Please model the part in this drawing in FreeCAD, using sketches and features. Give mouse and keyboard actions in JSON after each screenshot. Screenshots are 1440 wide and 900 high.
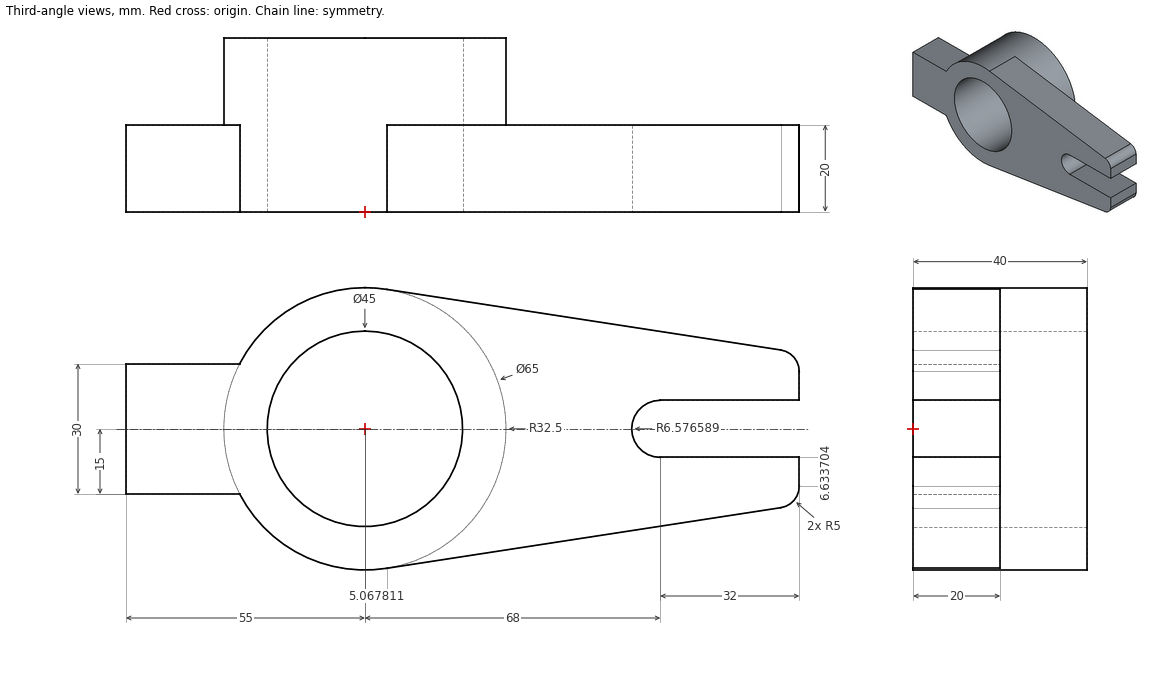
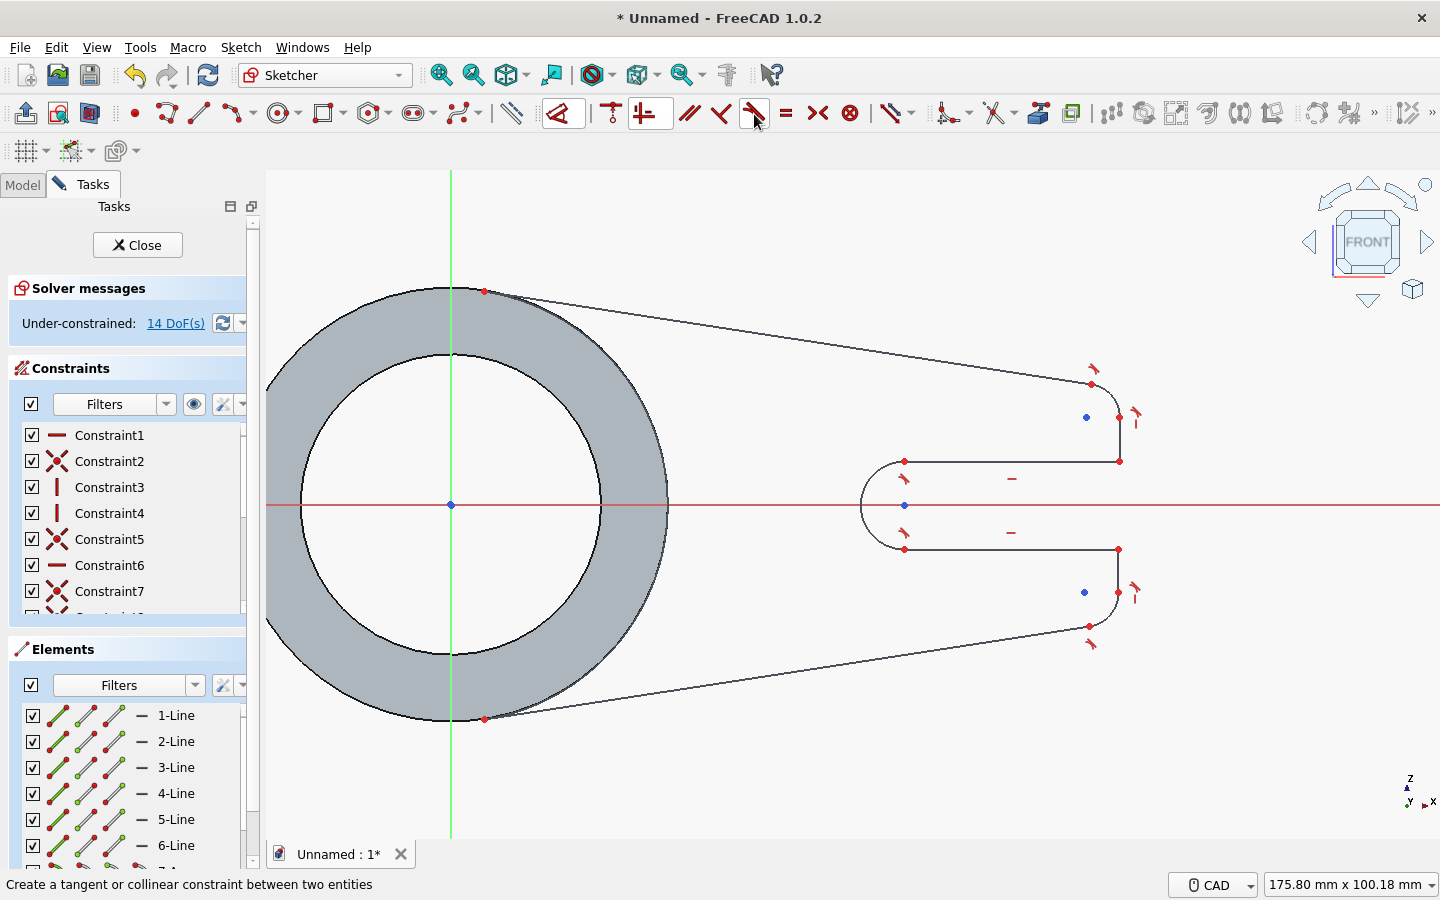
{"action": "left_click_drag", "start_coordinate": [441, 495], "coordinate": [461, 516]}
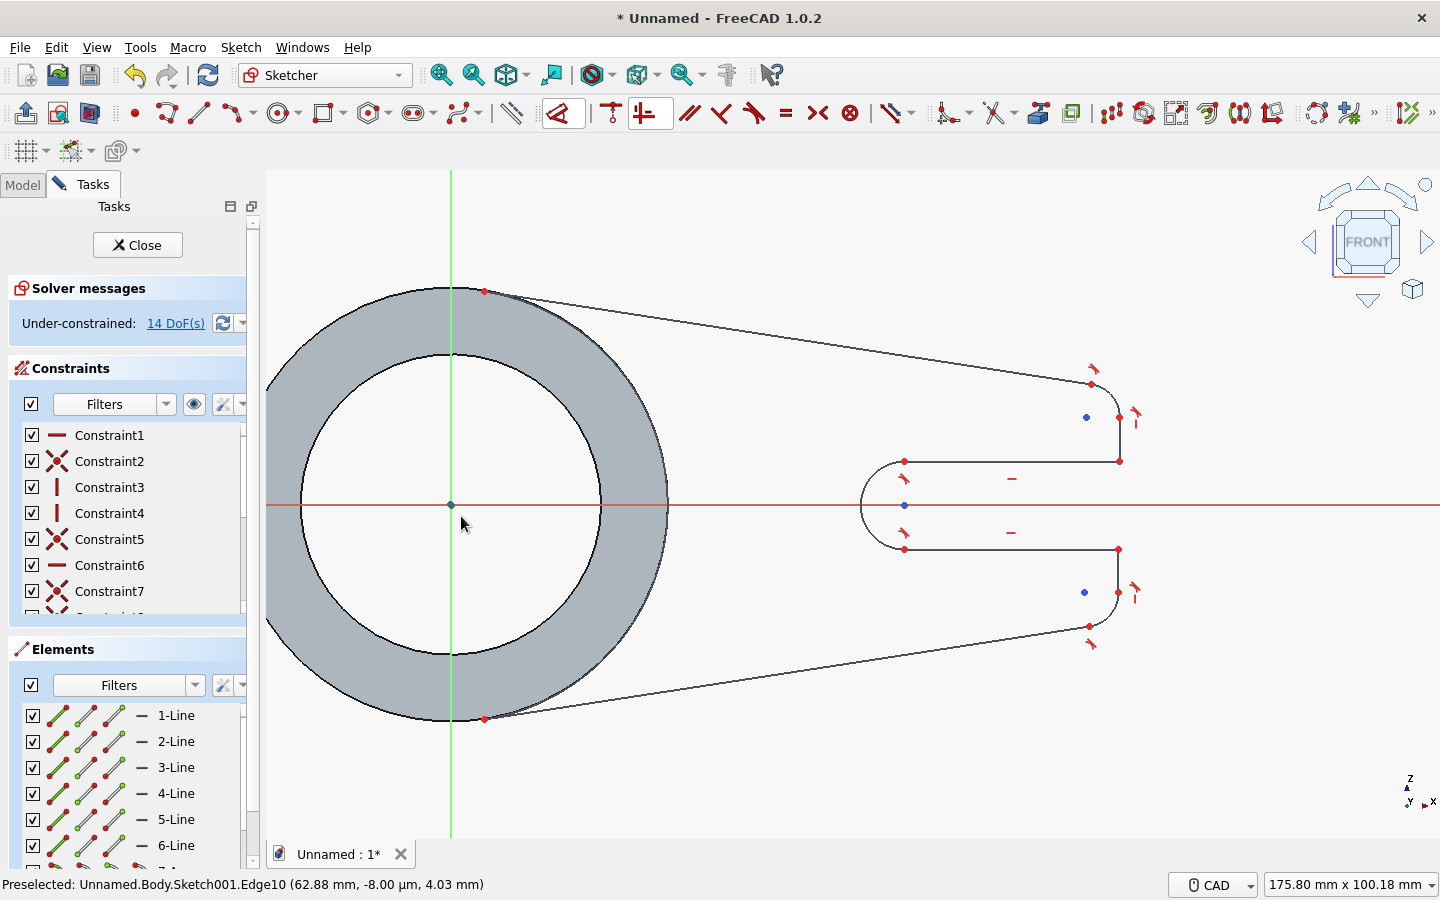
{"action": "left_click", "coordinate": [612, 114]}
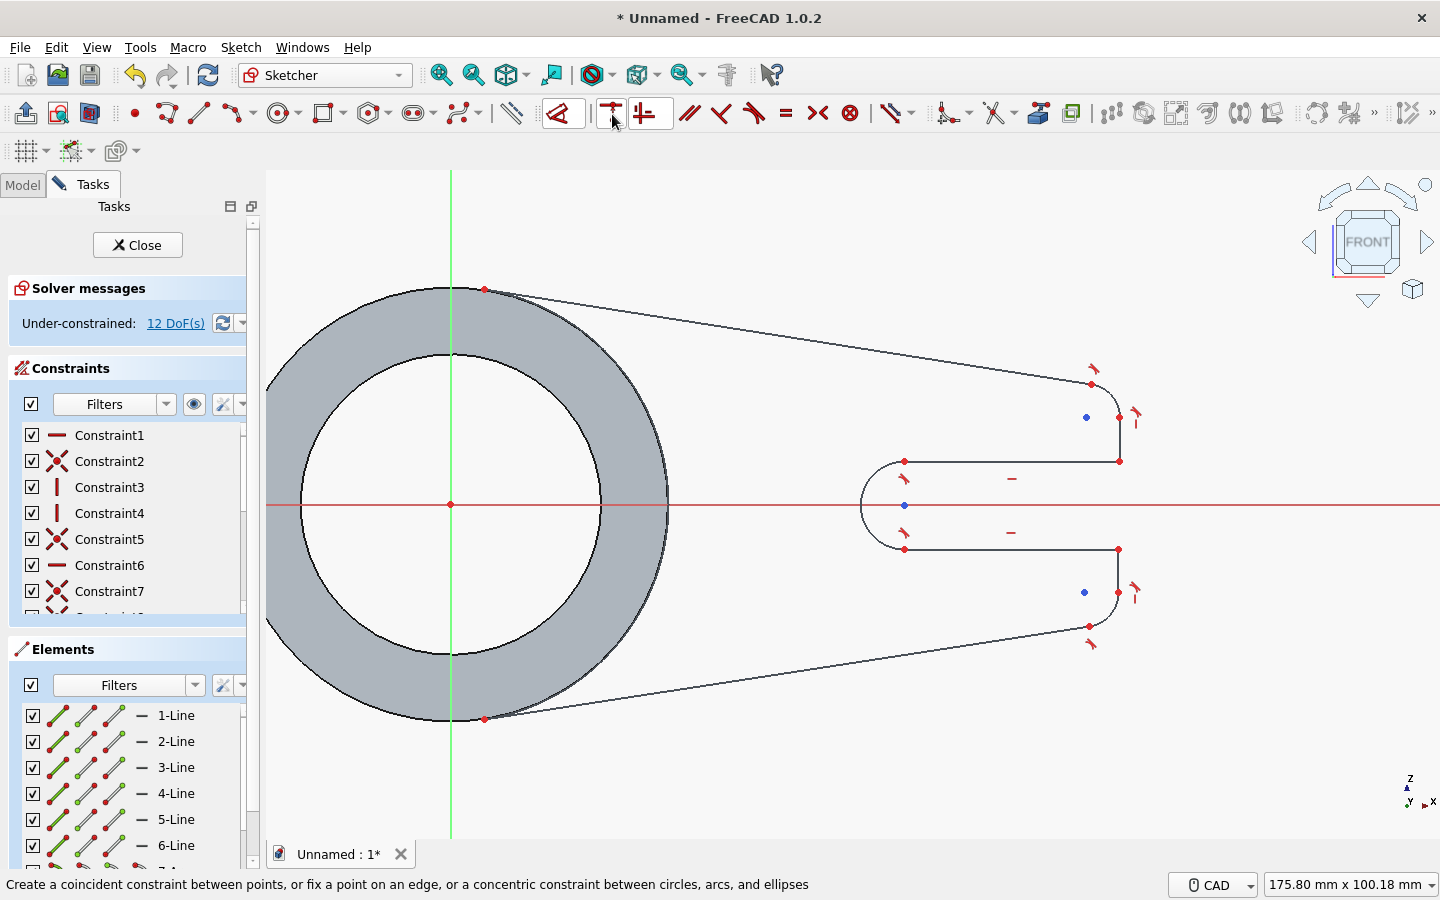
{"action": "left_click", "coordinate": [1103, 621]}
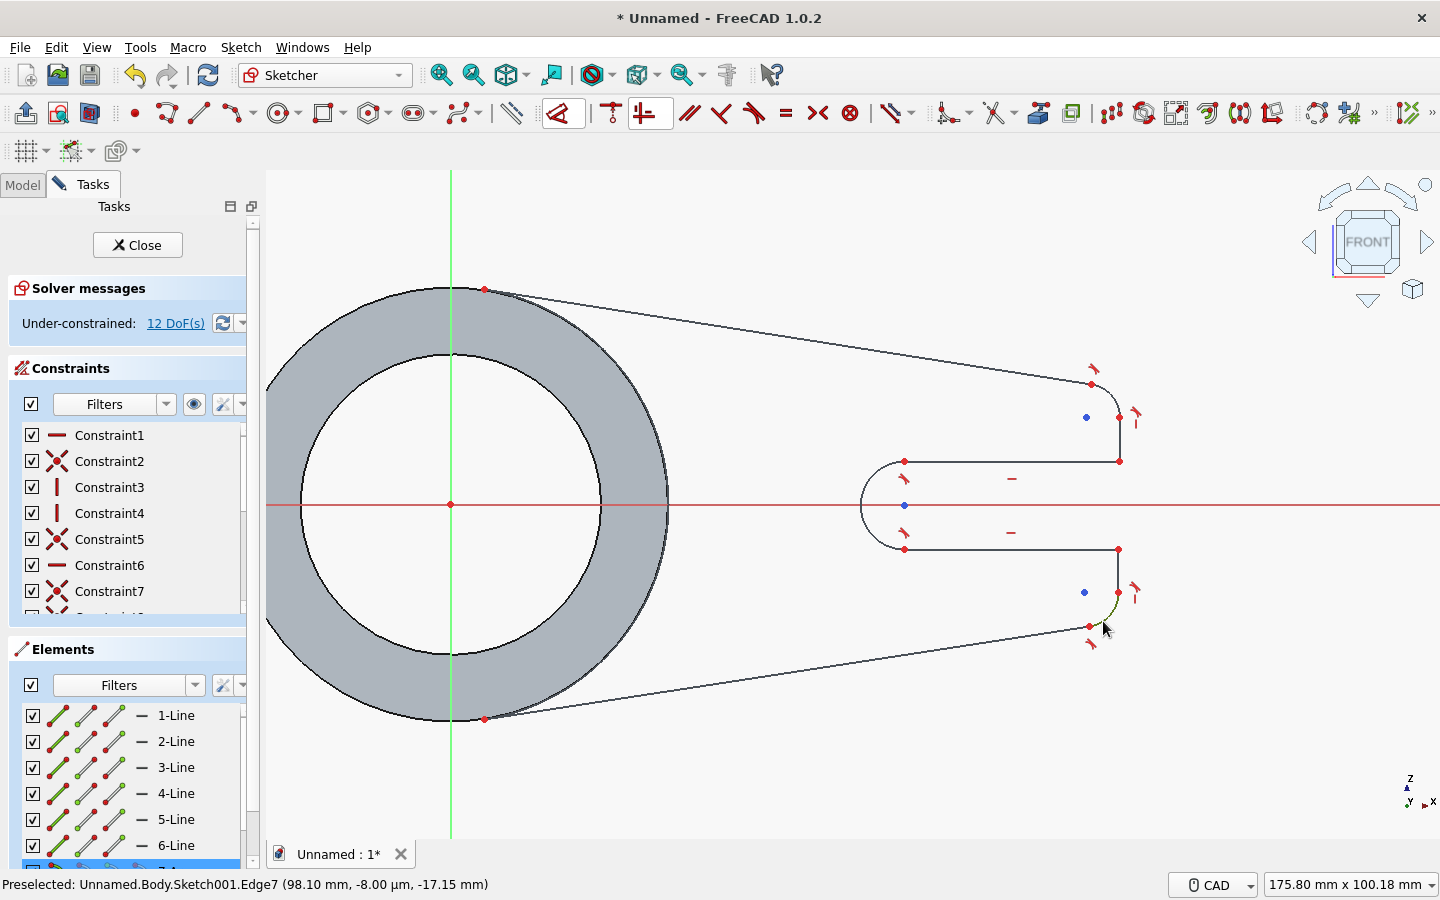
{"action": "left_click", "coordinate": [1117, 404]}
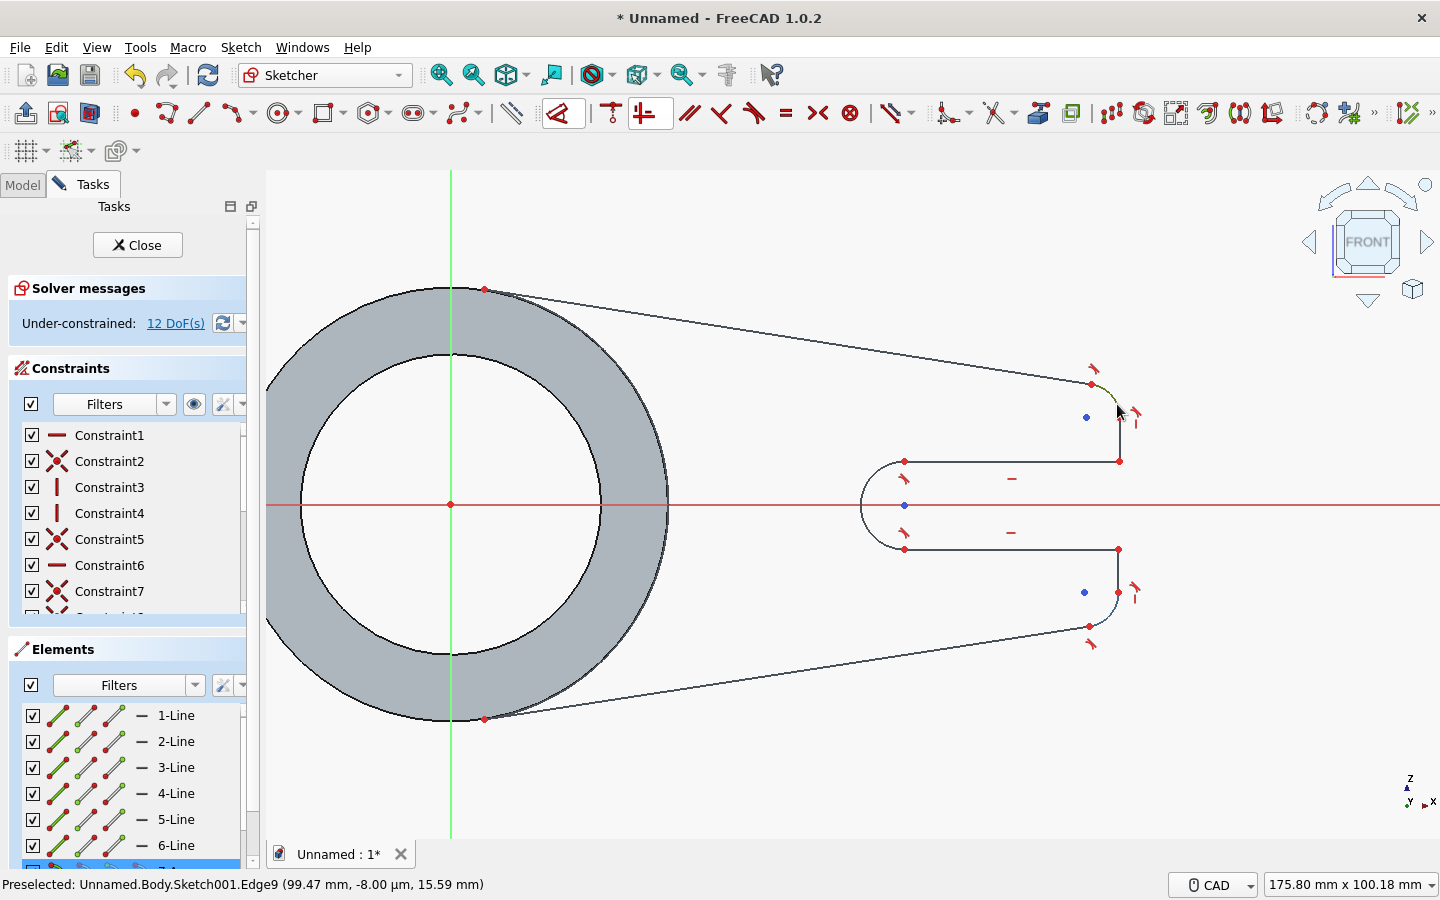
{"action": "left_click", "coordinate": [786, 114]}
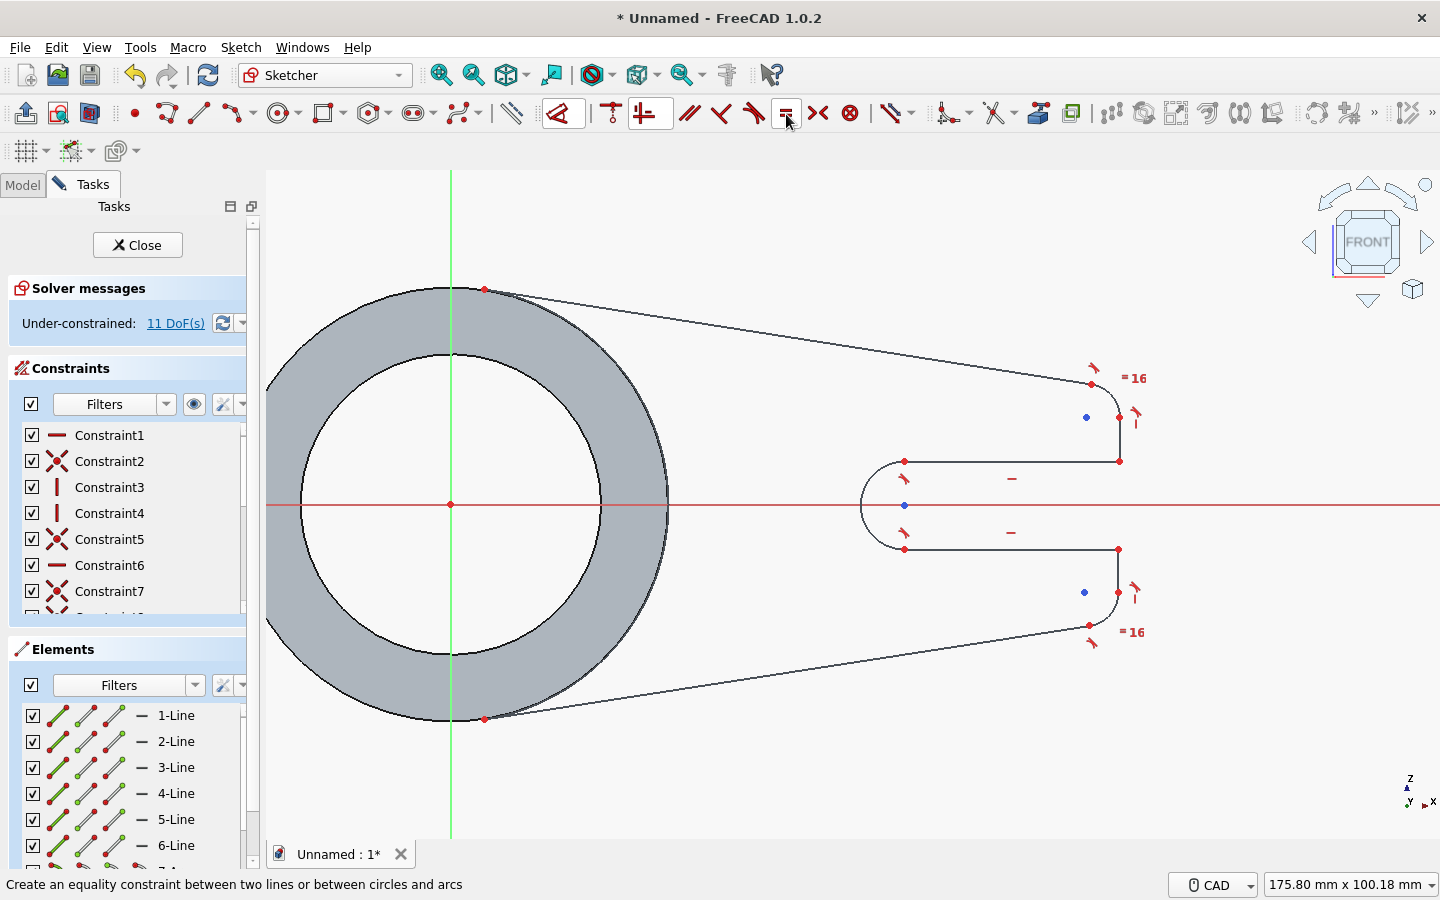
{"action": "left_click", "coordinate": [905, 506]}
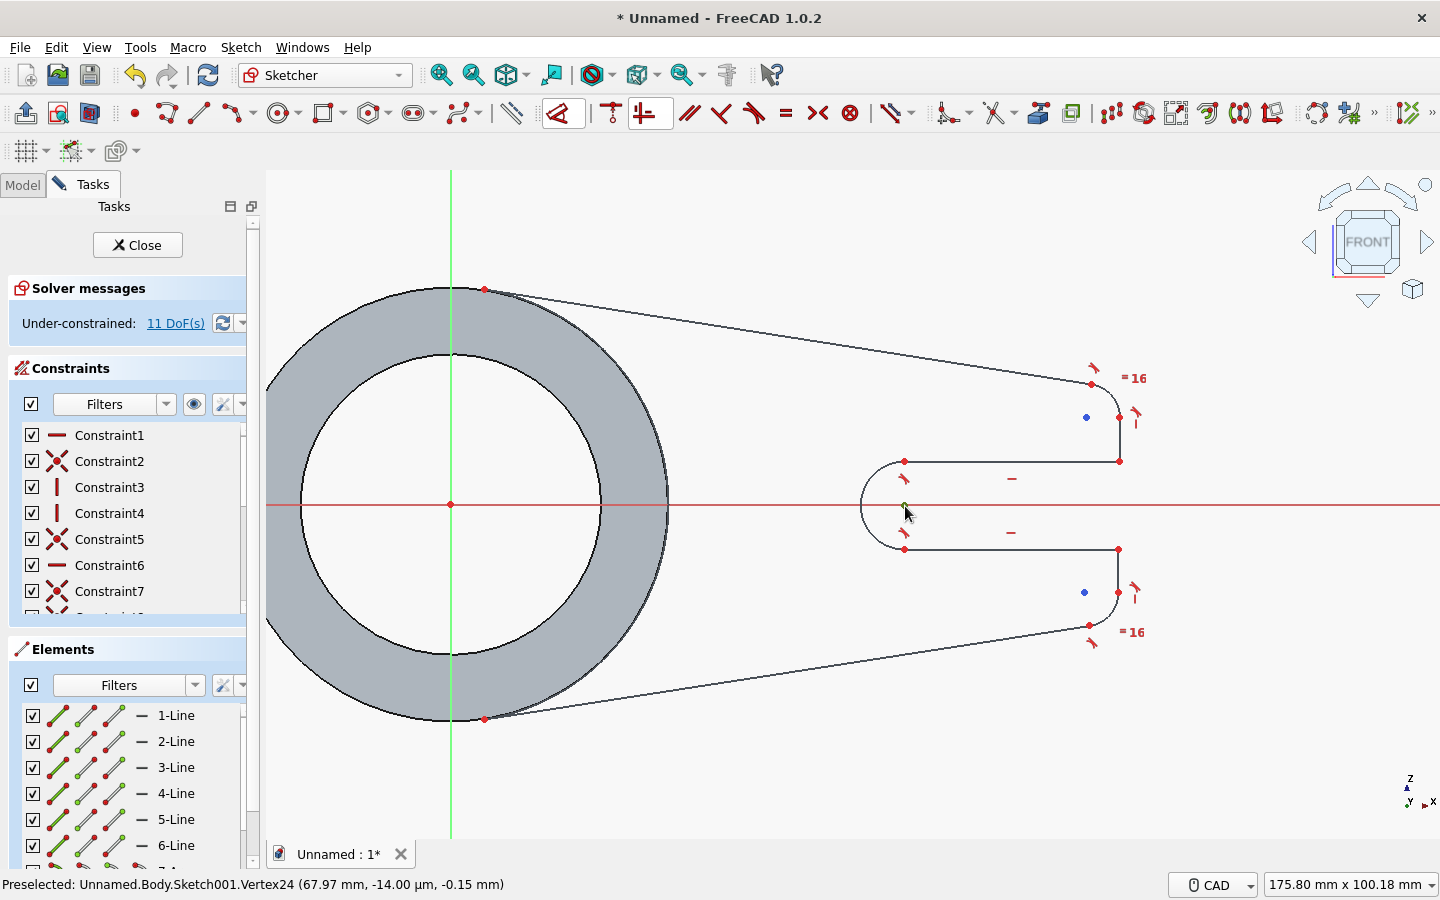
{"action": "left_click", "coordinate": [364, 505]}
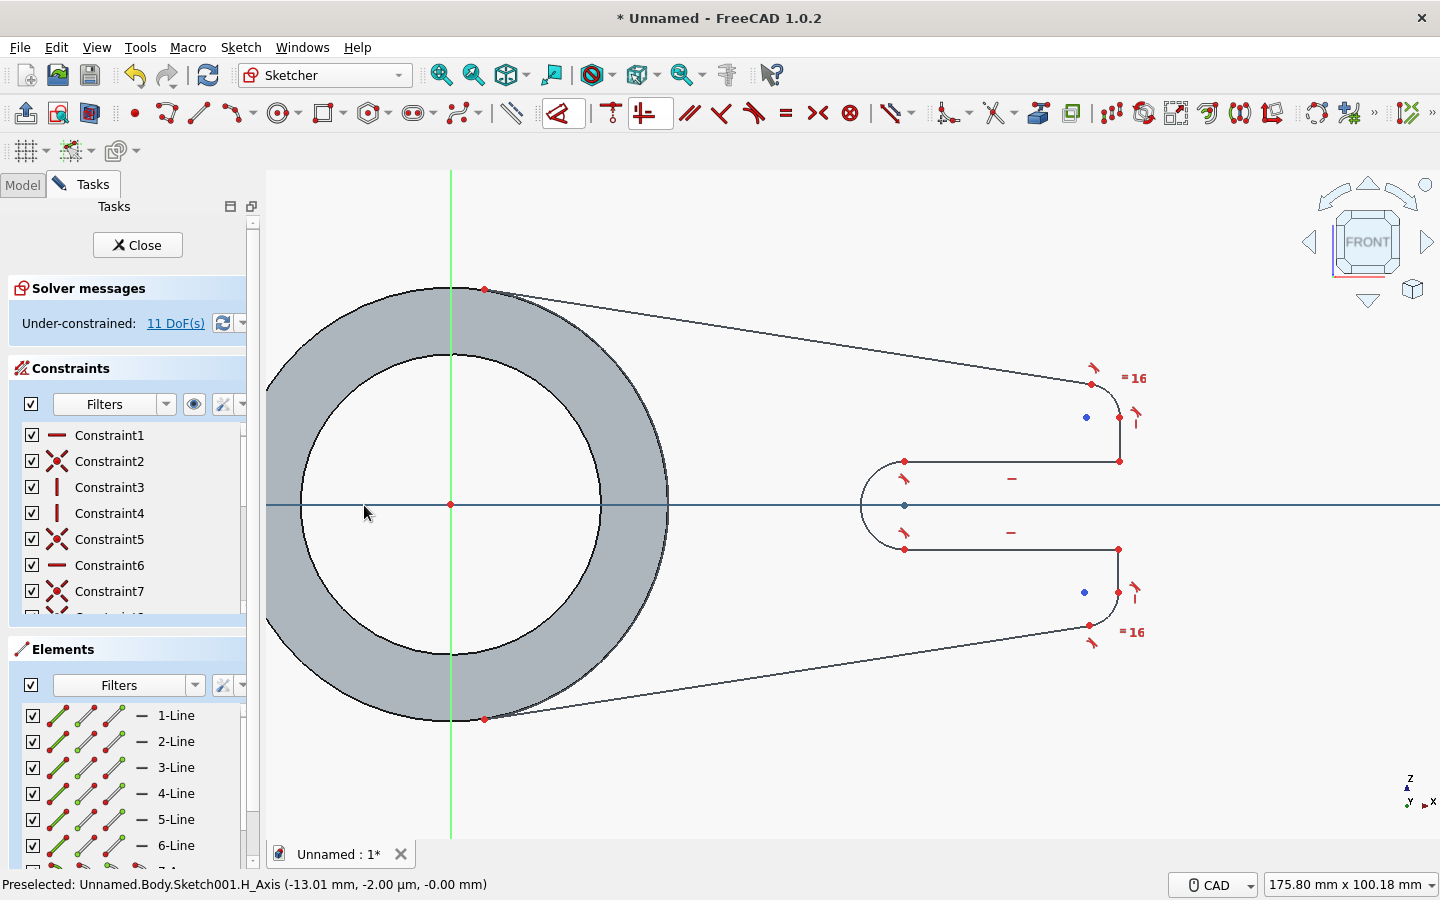
{"action": "left_click", "coordinate": [612, 114]}